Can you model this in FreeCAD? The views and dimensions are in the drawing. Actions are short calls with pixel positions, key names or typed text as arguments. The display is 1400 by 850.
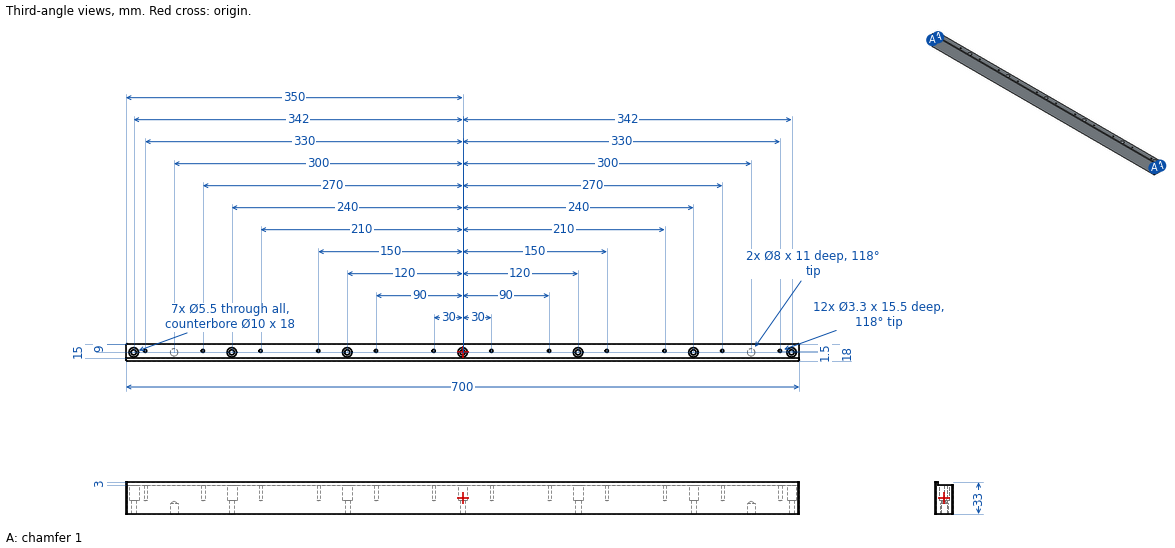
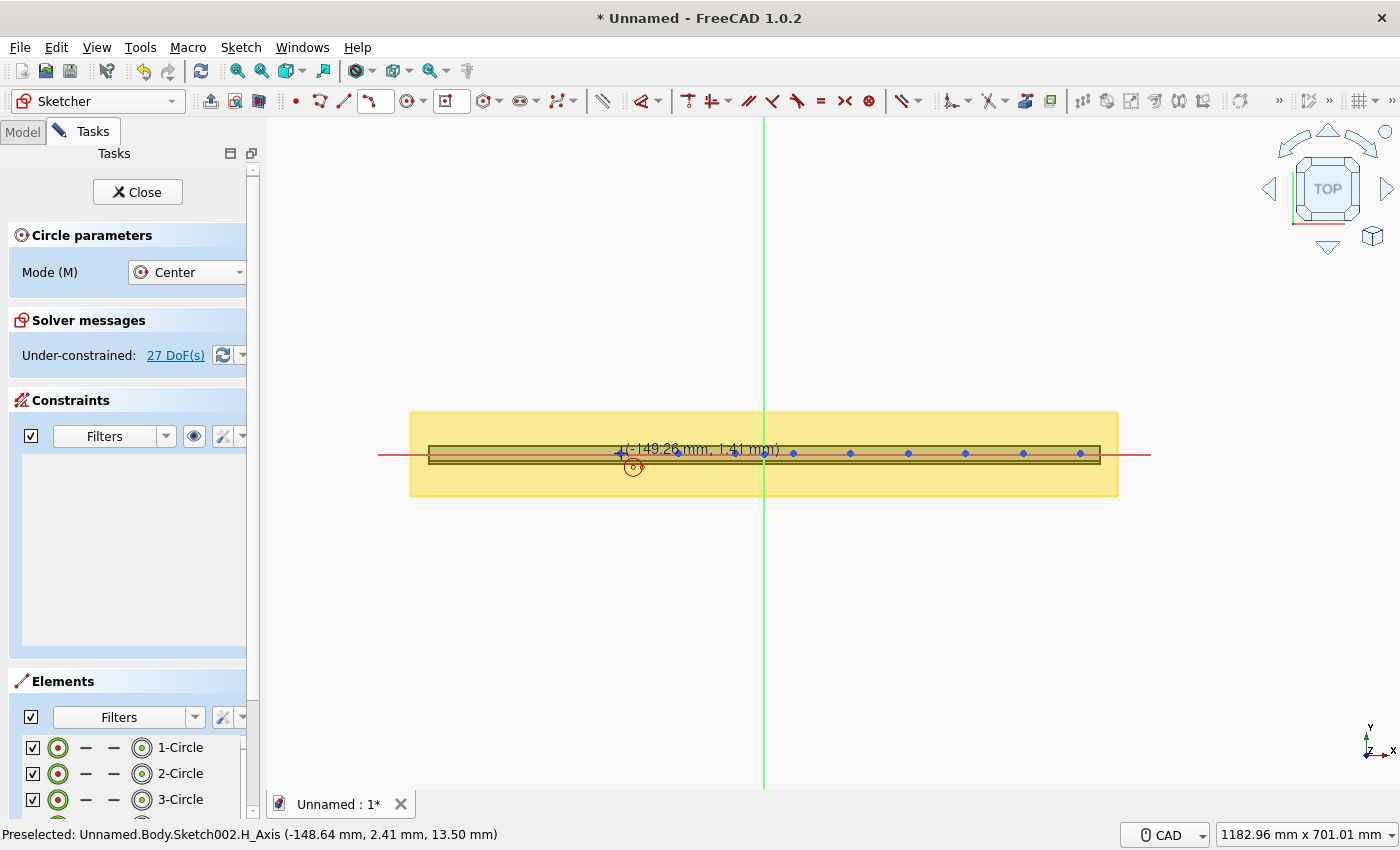
scroll(448, 453, up, 14)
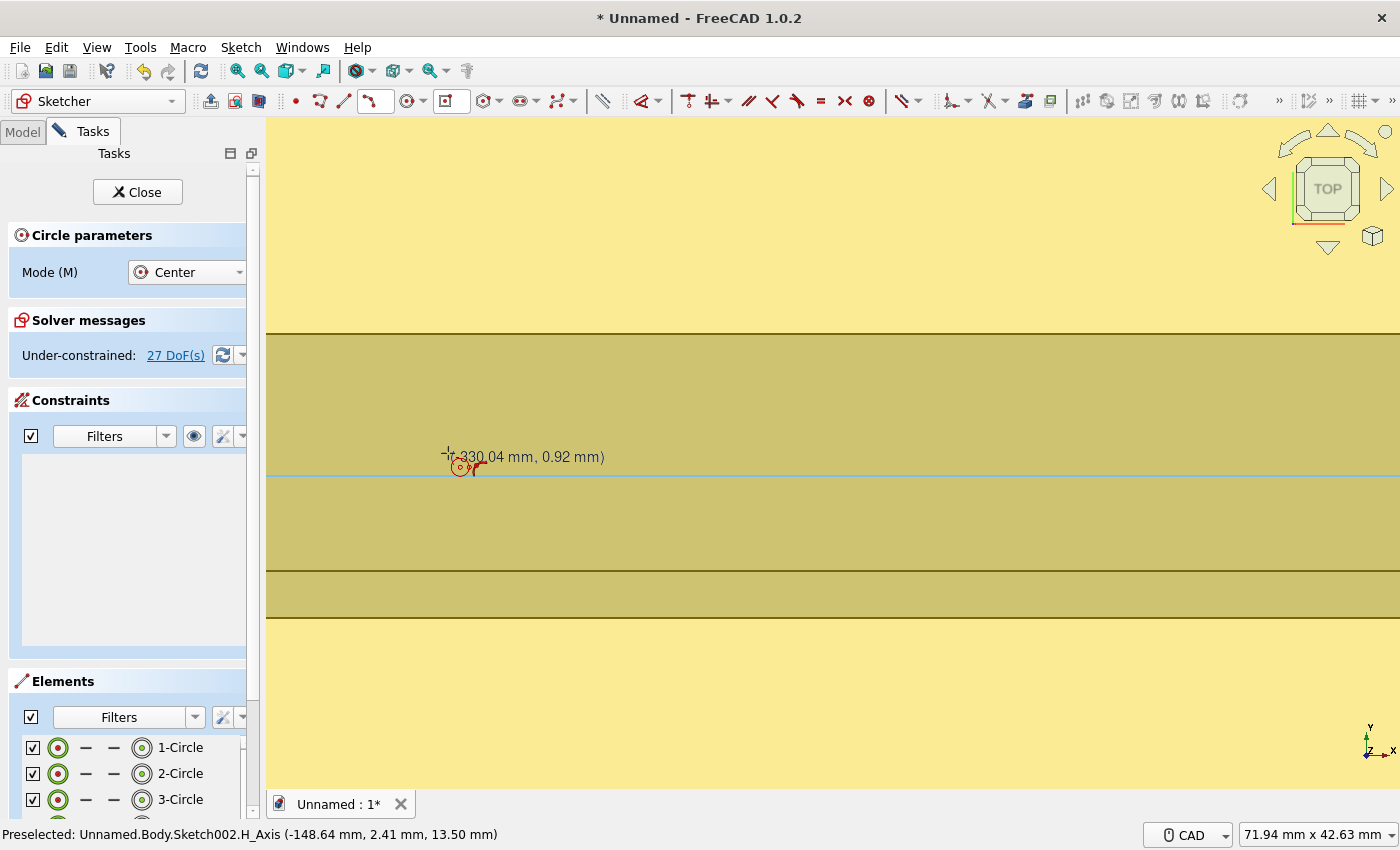
click(446, 453)
click(464, 434)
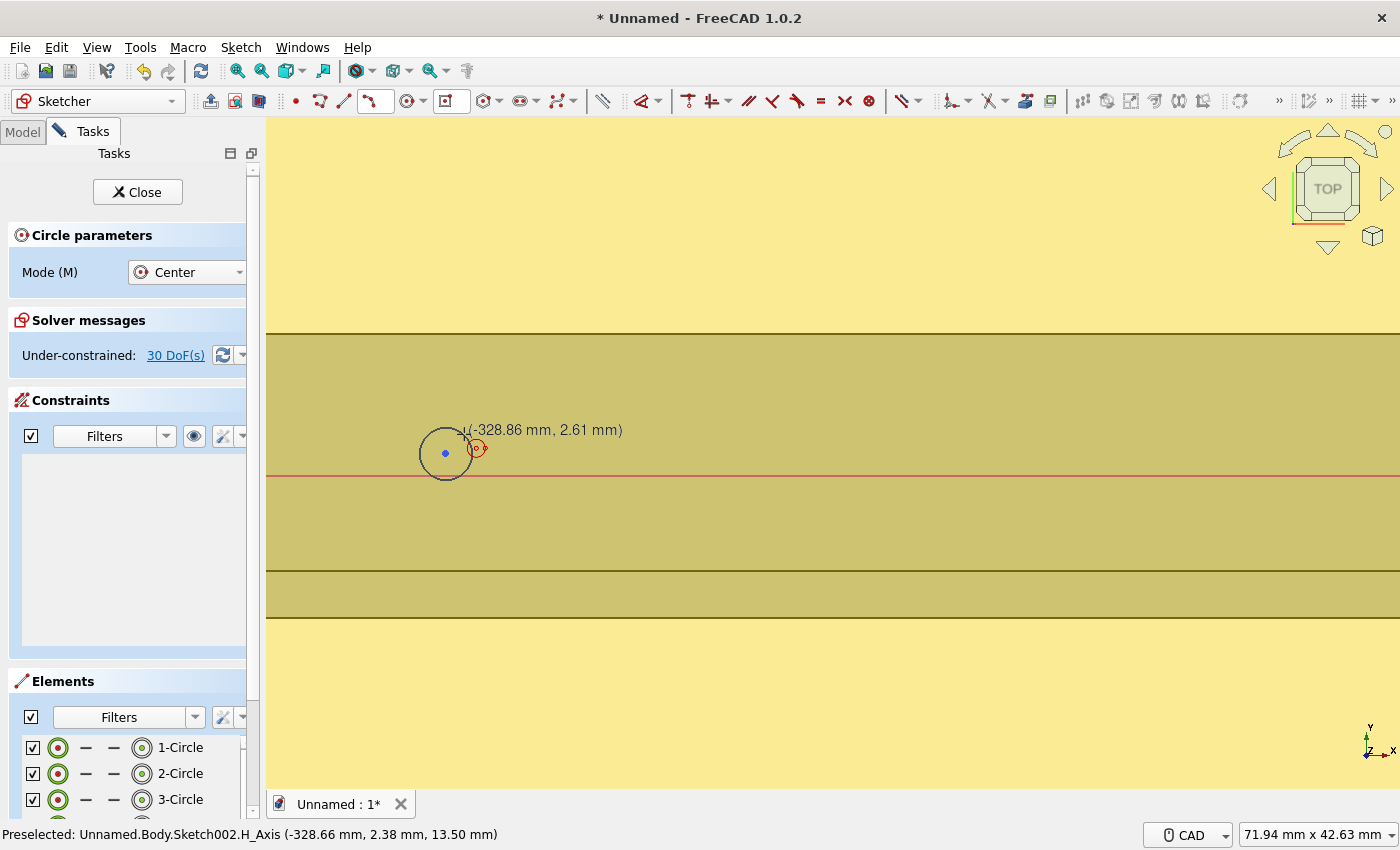
scroll(448, 453, down, 14)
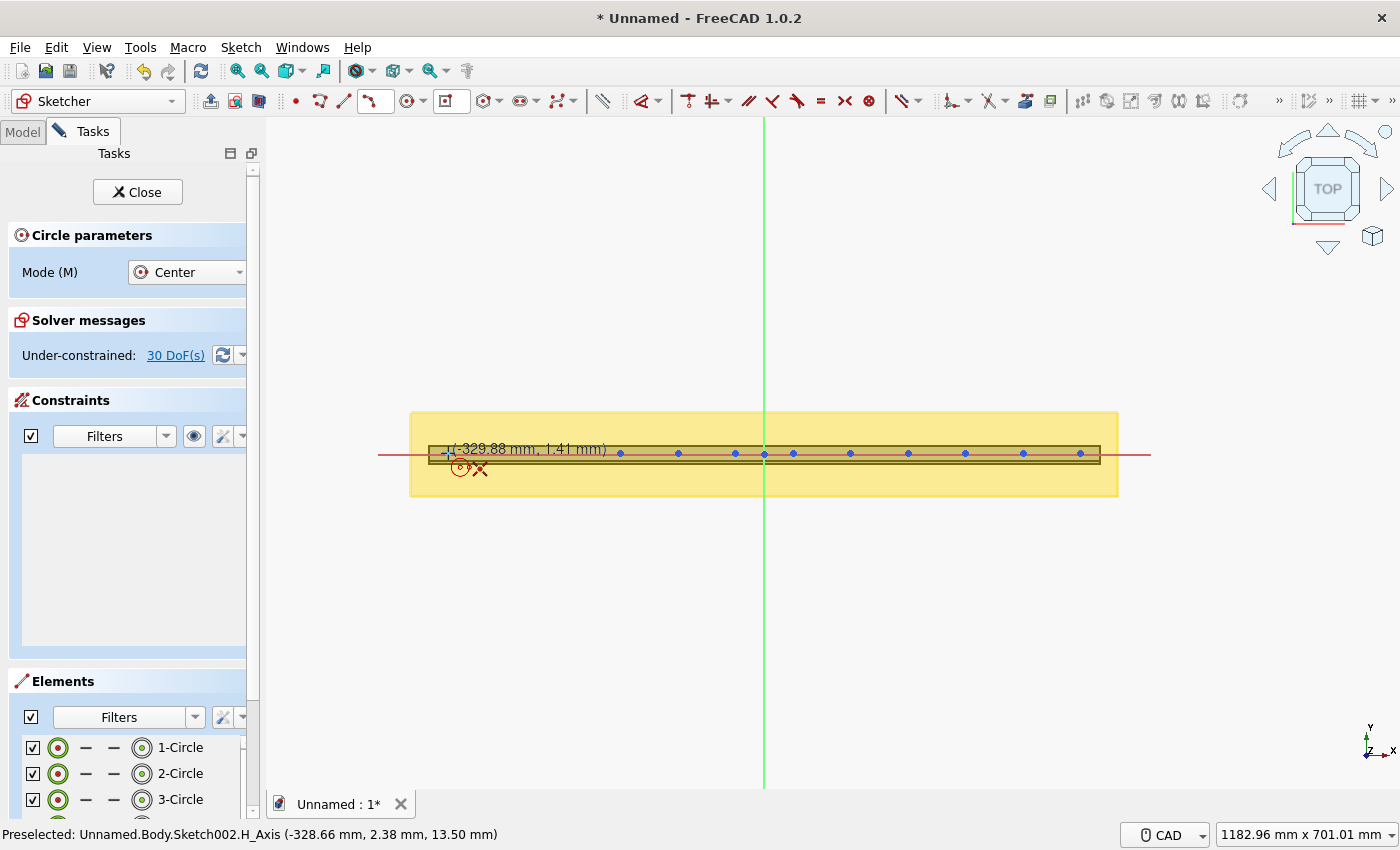
scroll(563, 453, up, 14)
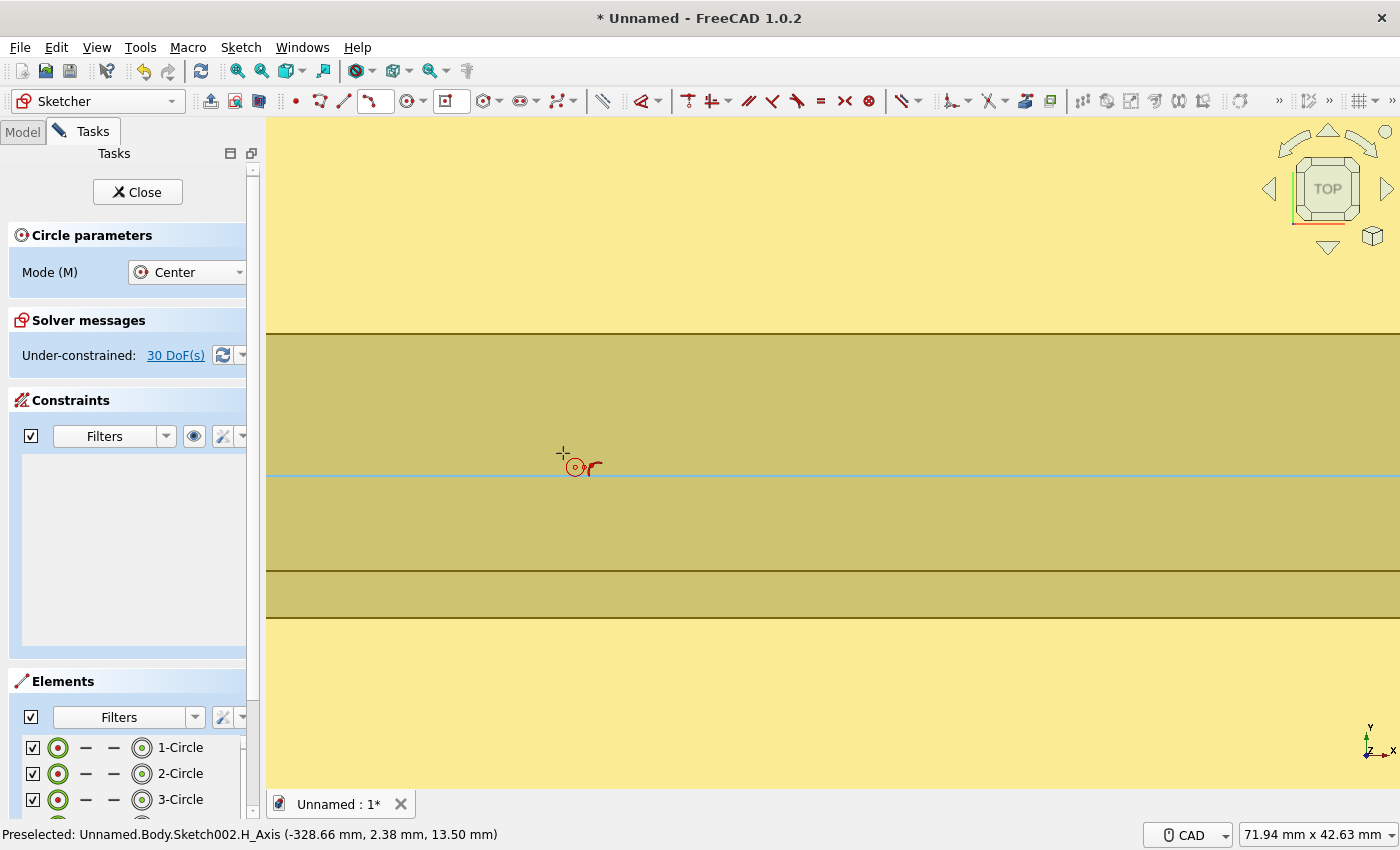
click(560, 453)
click(578, 434)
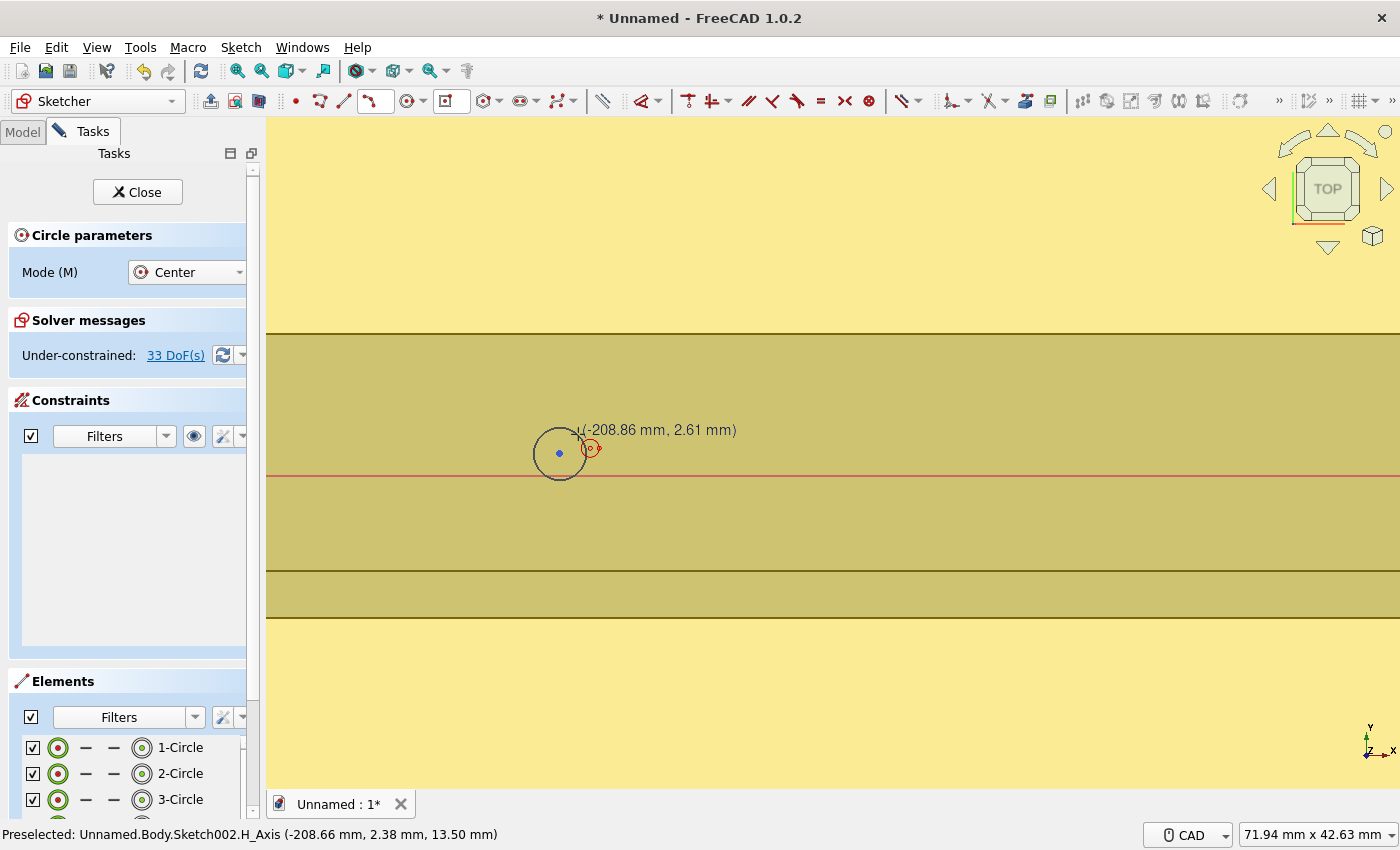
scroll(563, 453, down, 14)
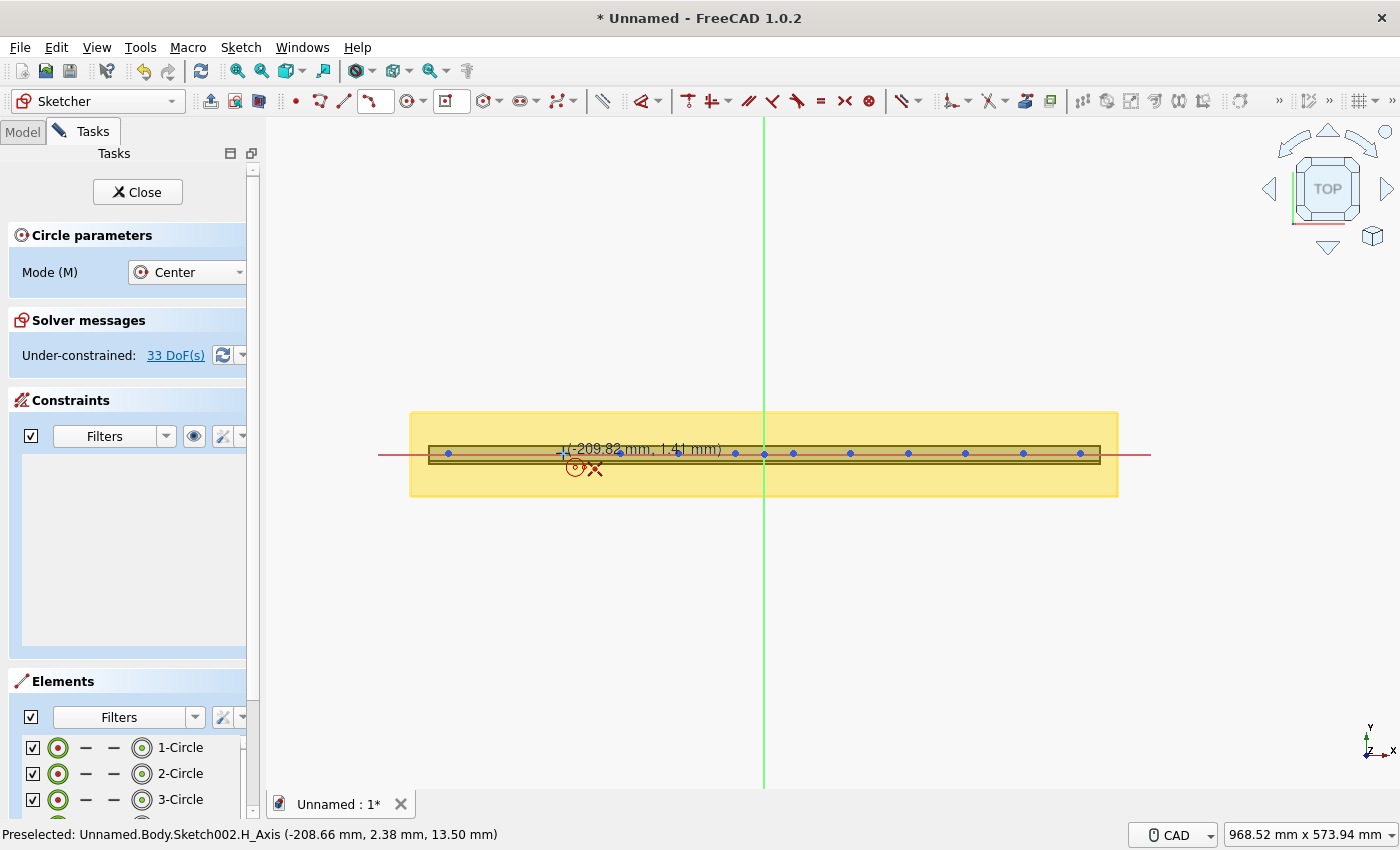
scroll(506, 453, up, 14)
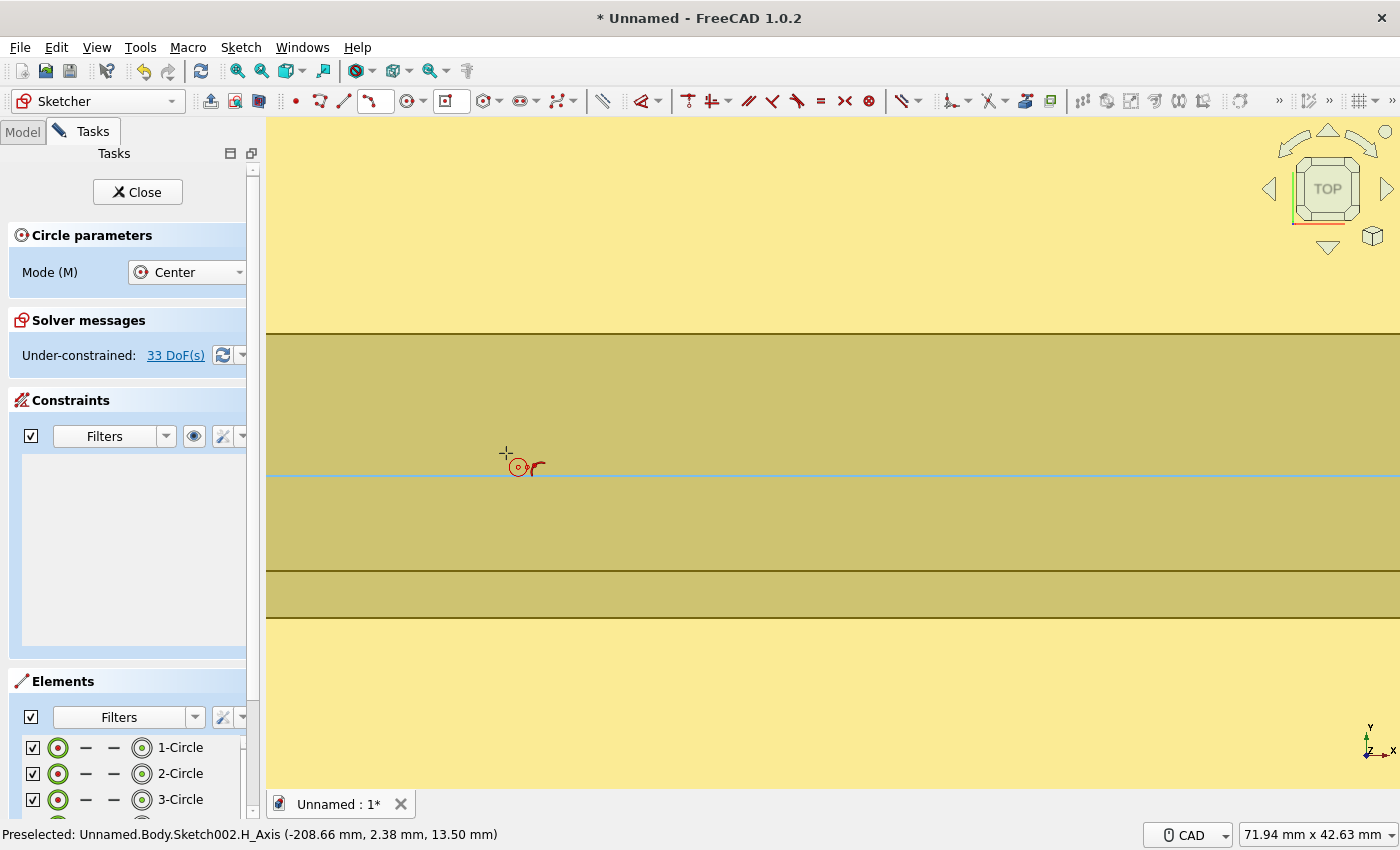
click(495, 453)
click(514, 434)
key(Escape)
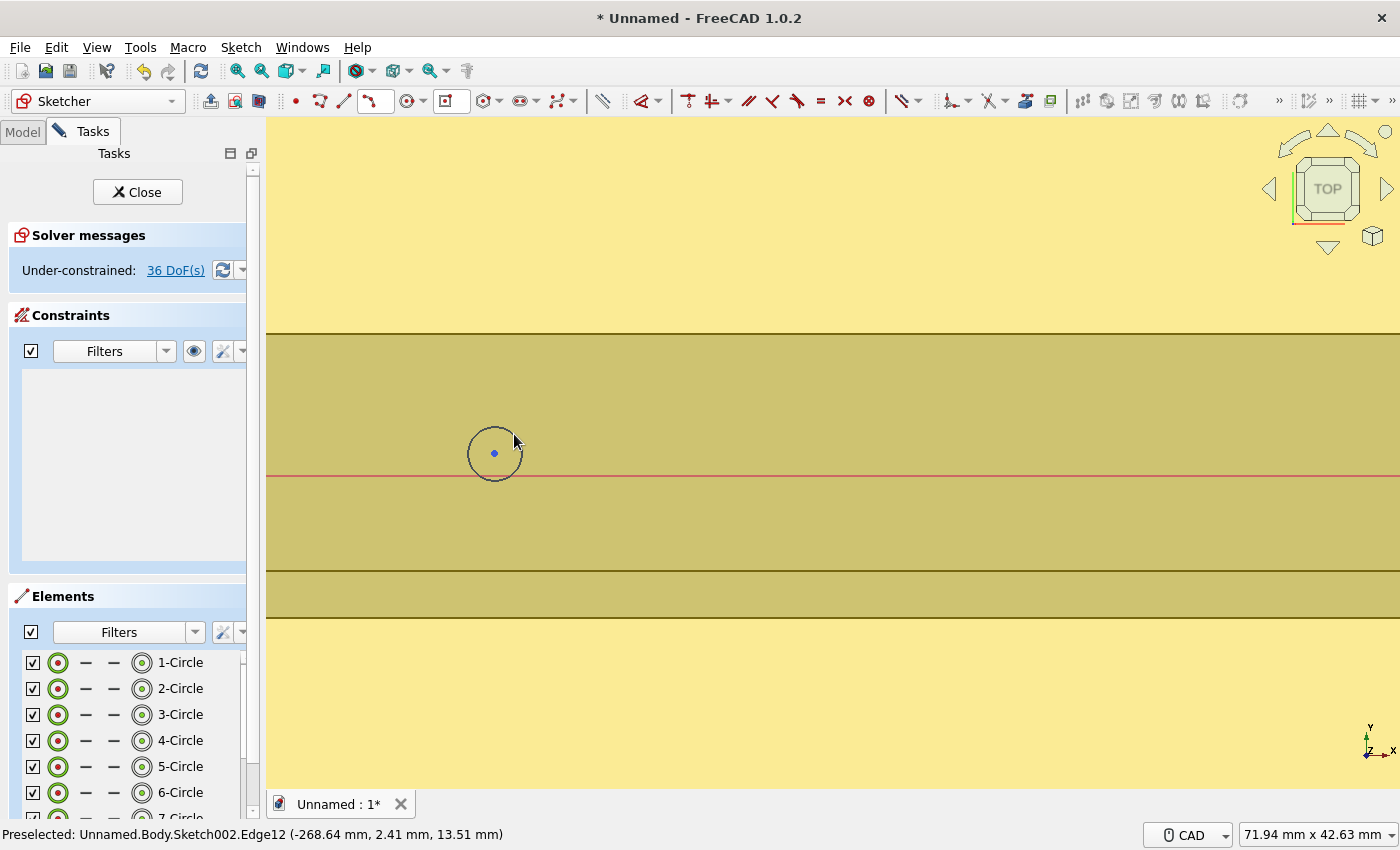
scroll(506, 453, down, 14)